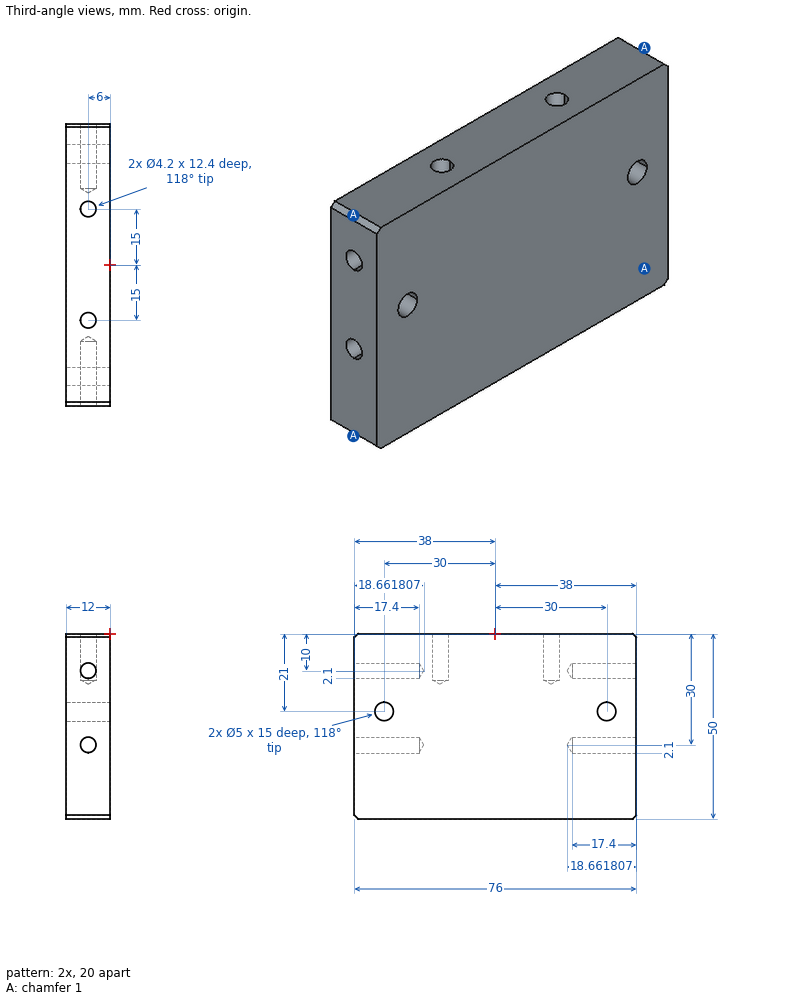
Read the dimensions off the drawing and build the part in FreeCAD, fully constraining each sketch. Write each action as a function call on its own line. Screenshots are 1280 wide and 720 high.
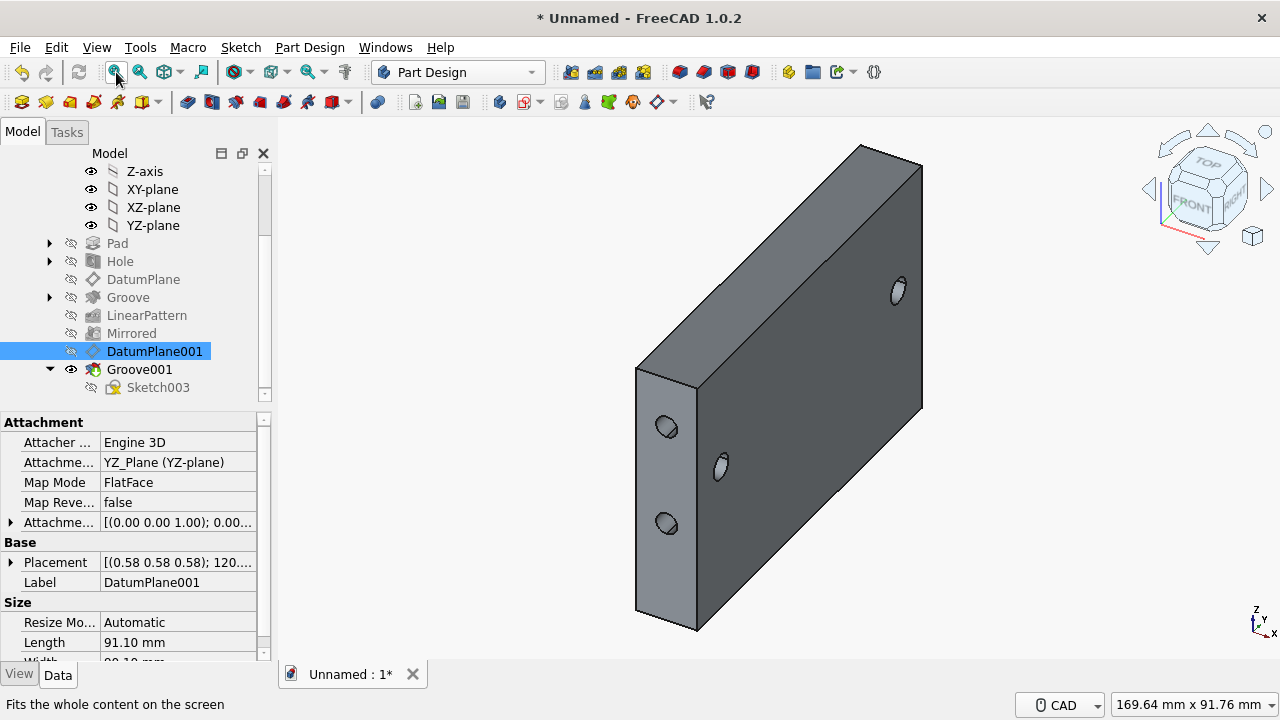
click(318, 619)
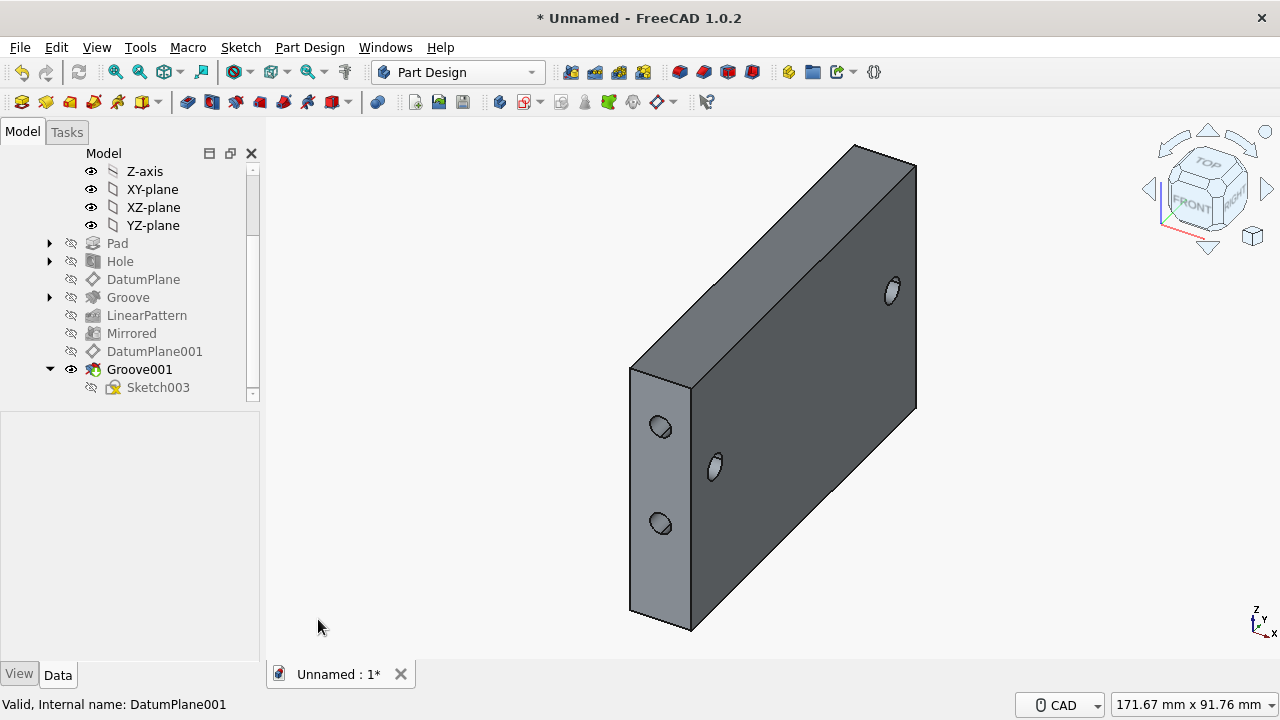
click(524, 102)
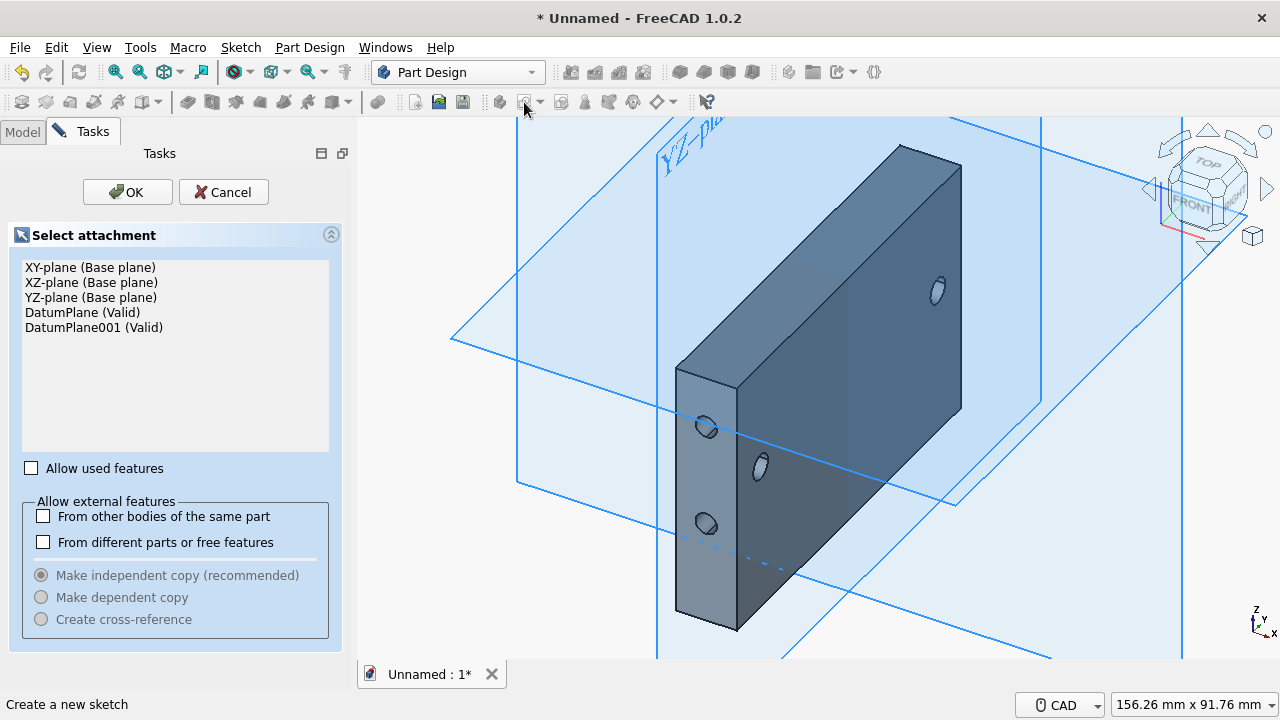
click(82, 268)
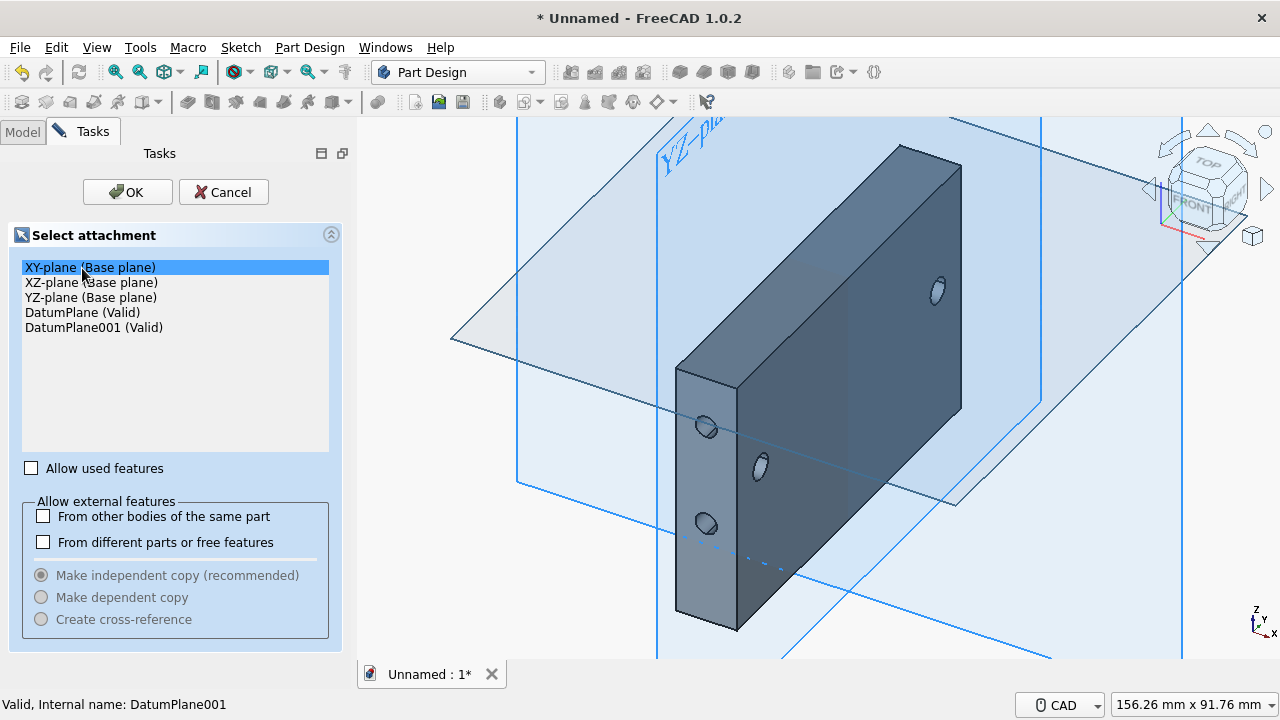
click(128, 192)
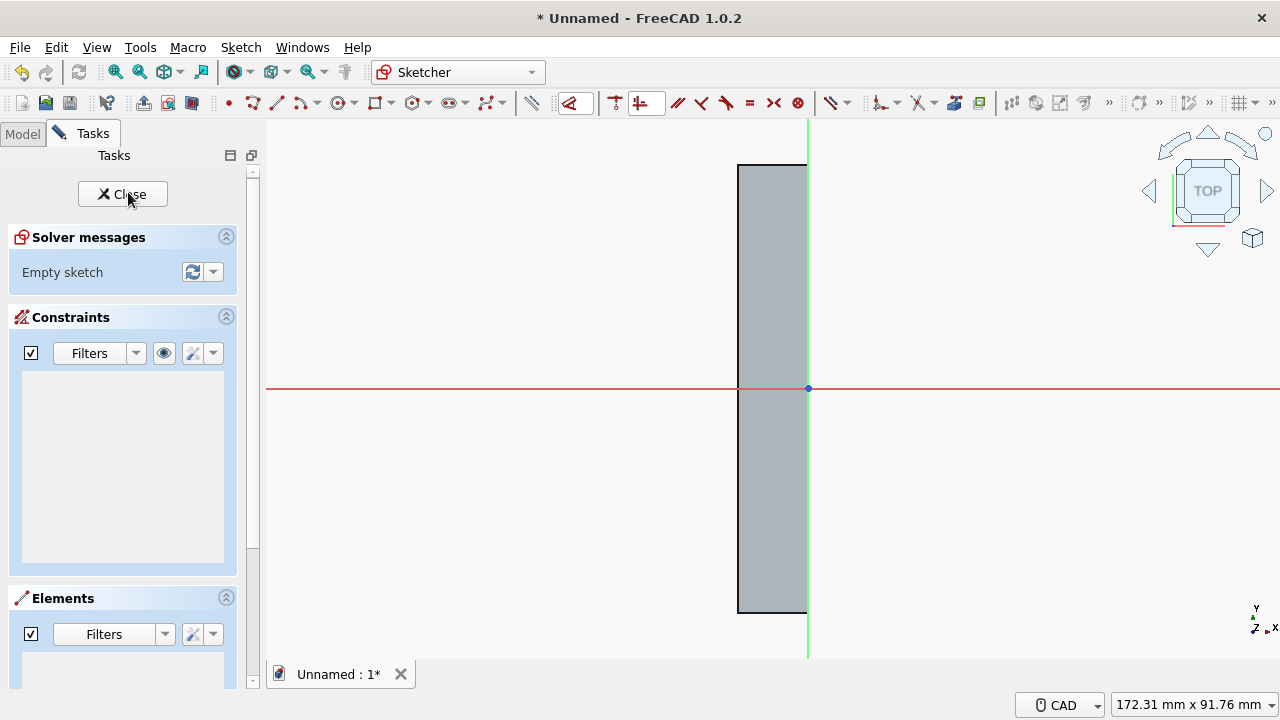
scroll(882, 389, up, 3)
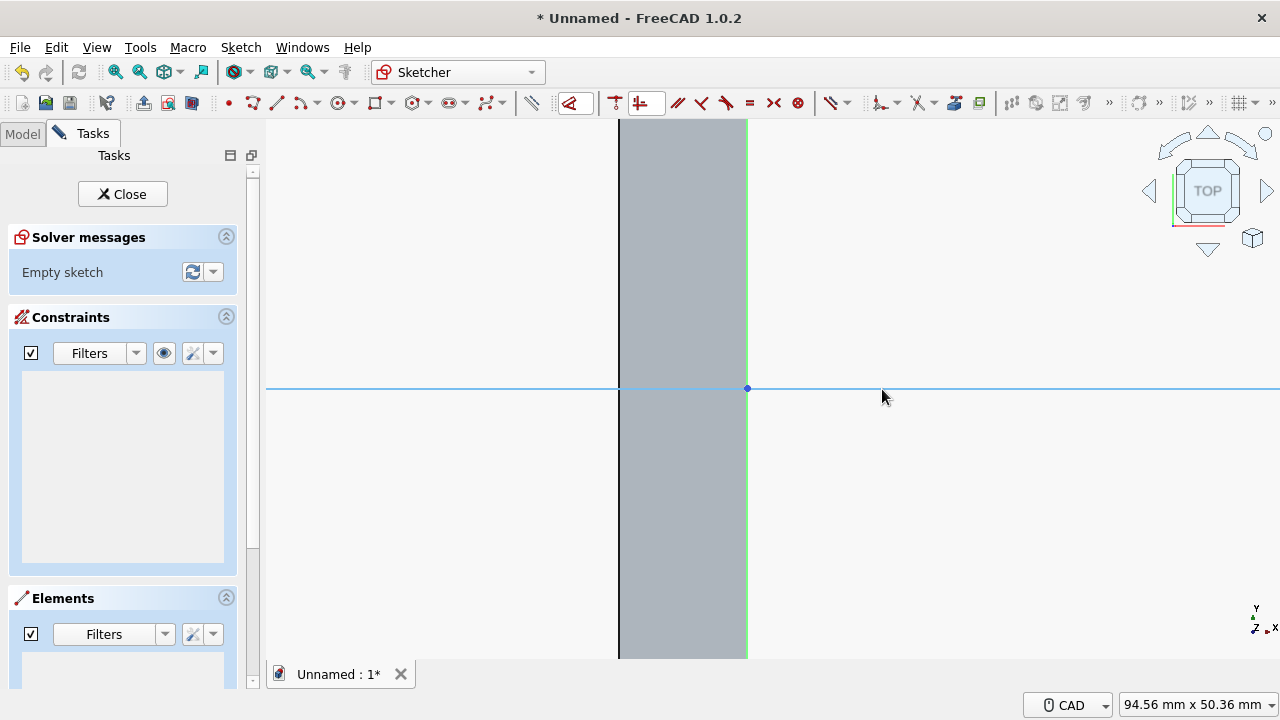
click(338, 104)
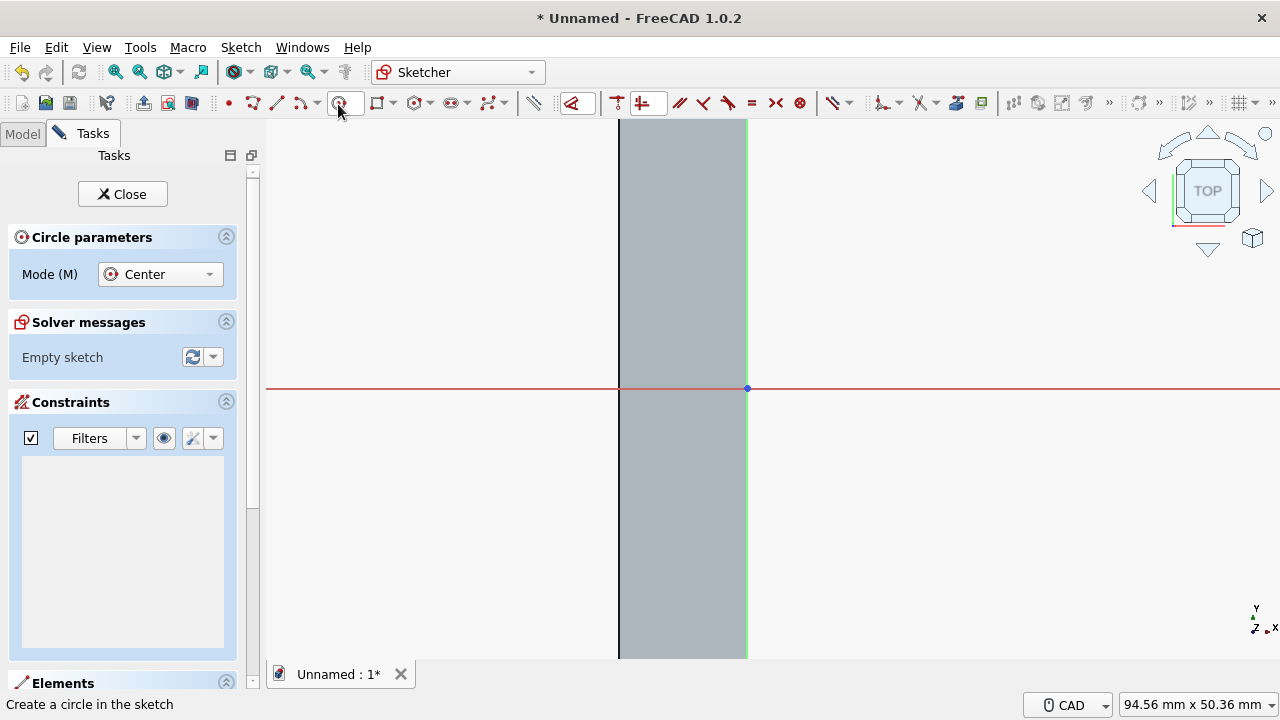
click(683, 228)
move(699, 212)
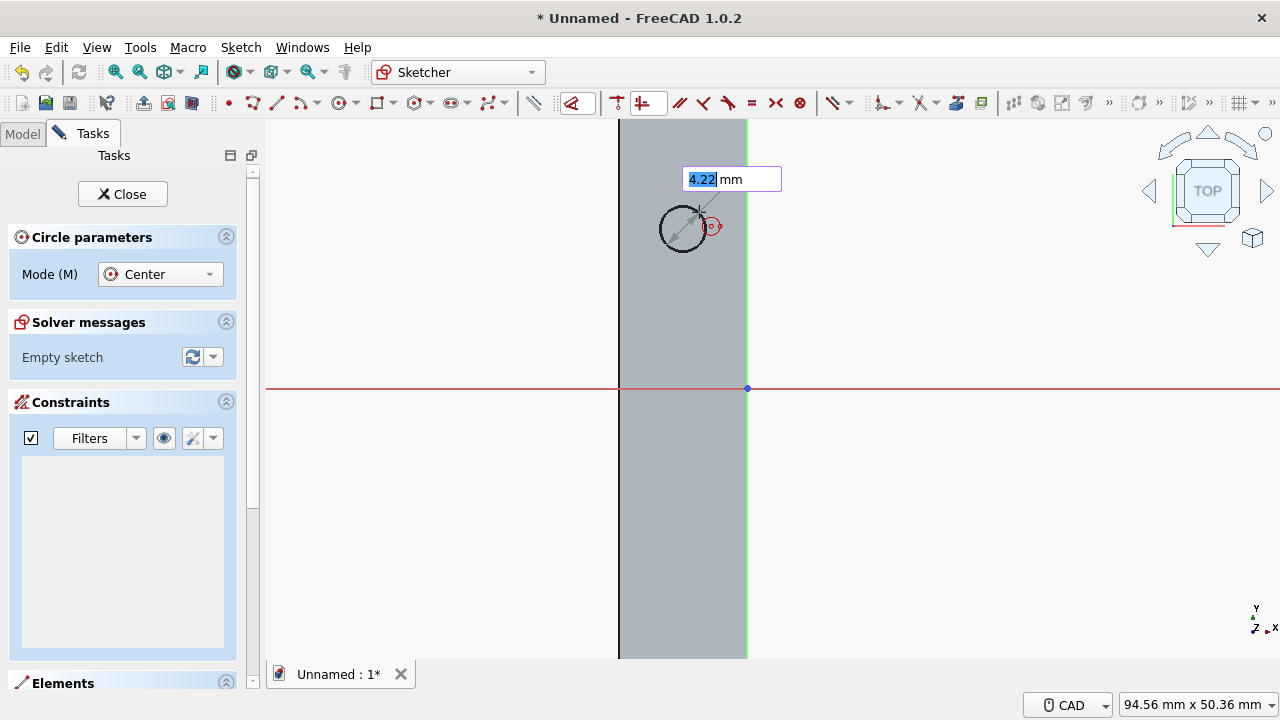
text(4.2)
key(Return)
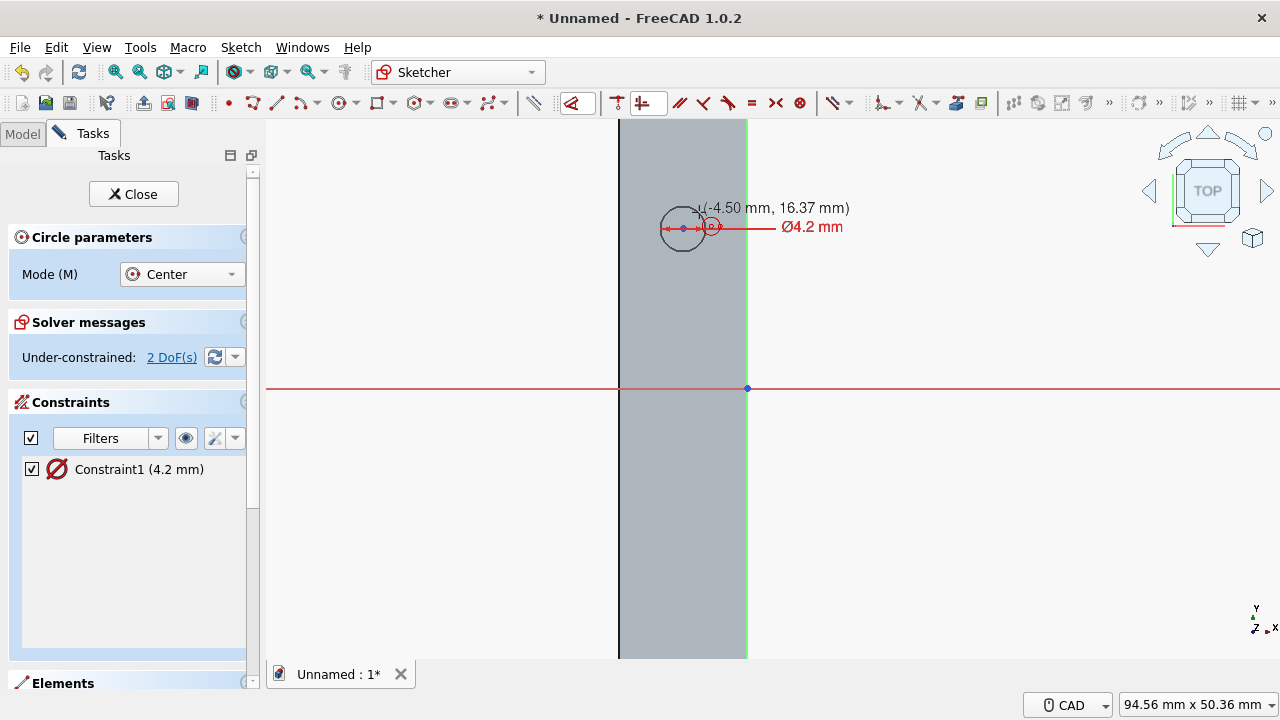
click(683, 549)
move(699, 534)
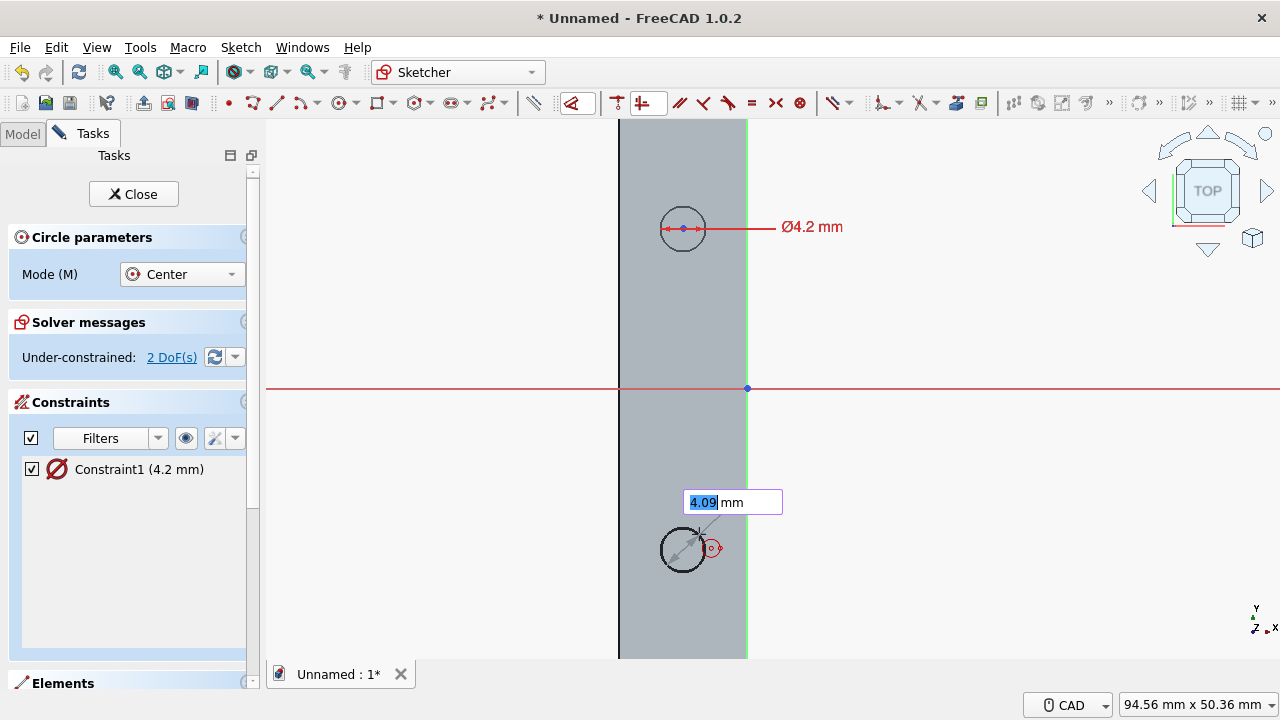
text(4.2)
key(Return)
key(Escape)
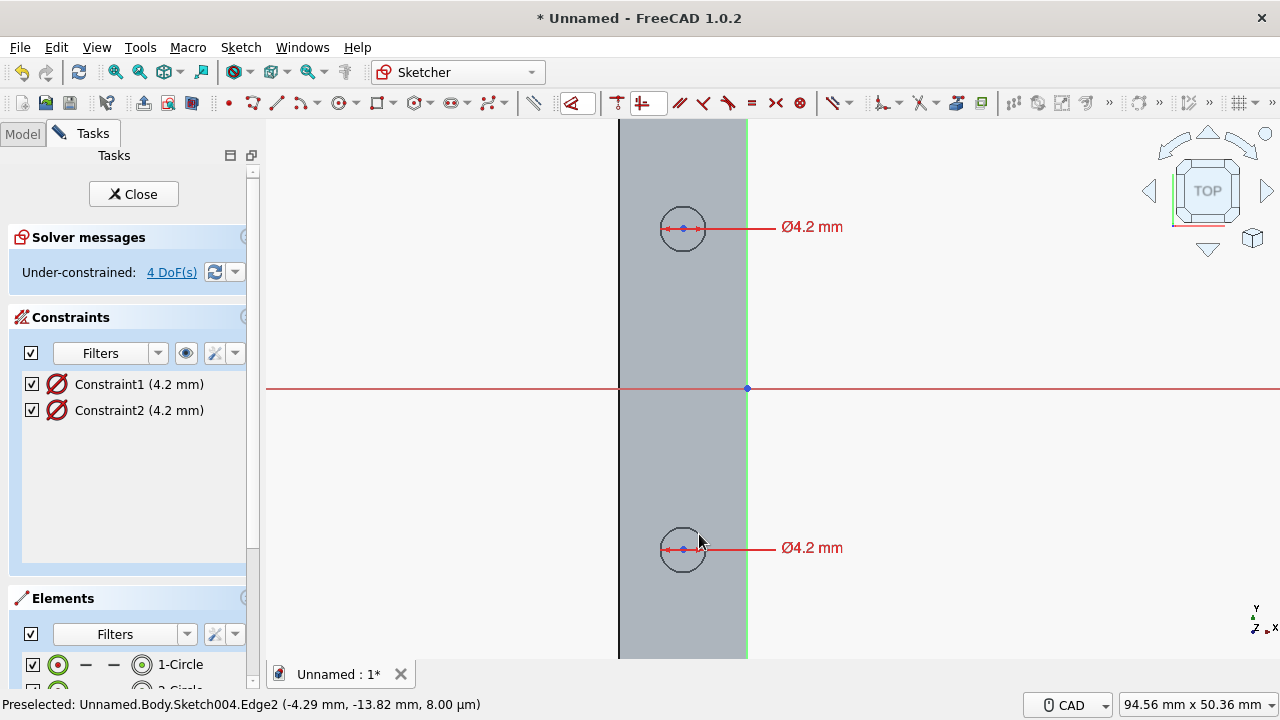
click(683, 229)